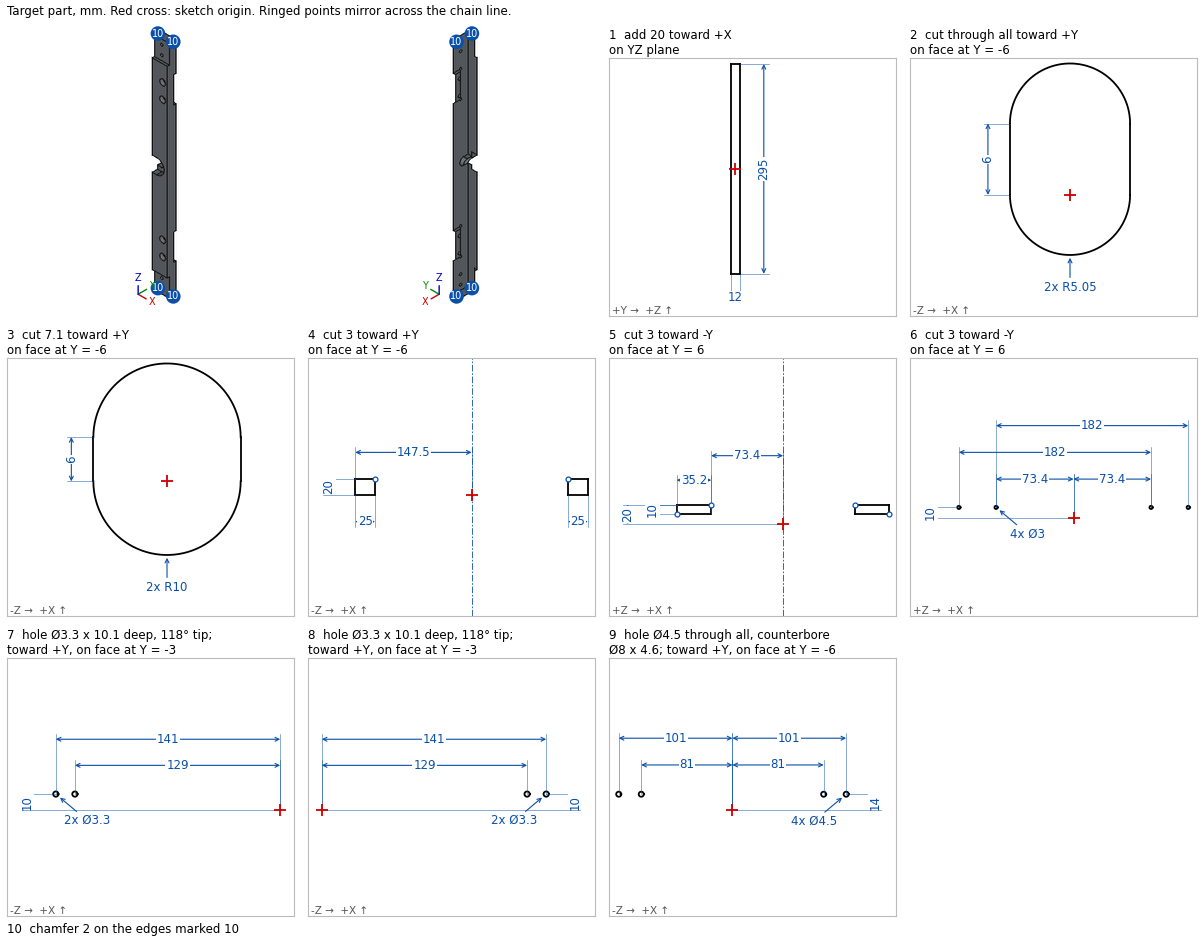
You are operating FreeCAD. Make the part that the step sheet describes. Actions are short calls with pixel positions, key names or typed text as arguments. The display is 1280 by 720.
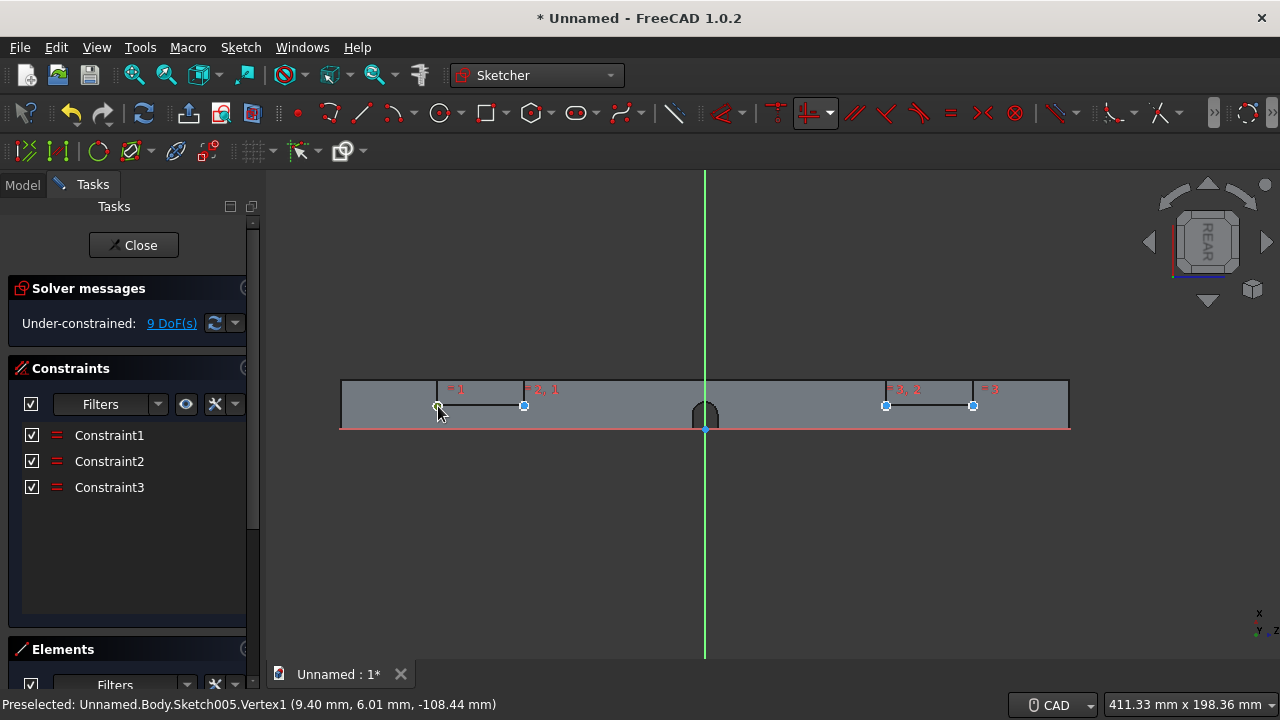
click(524, 406)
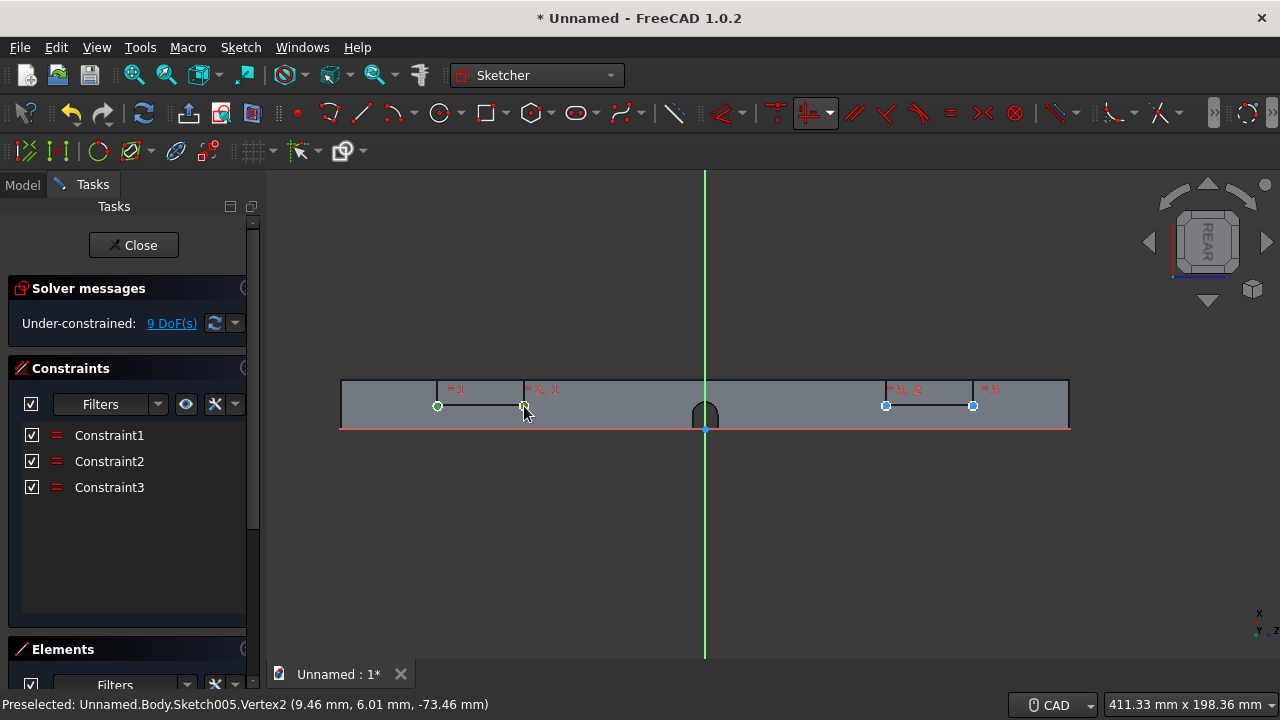
click(832, 114)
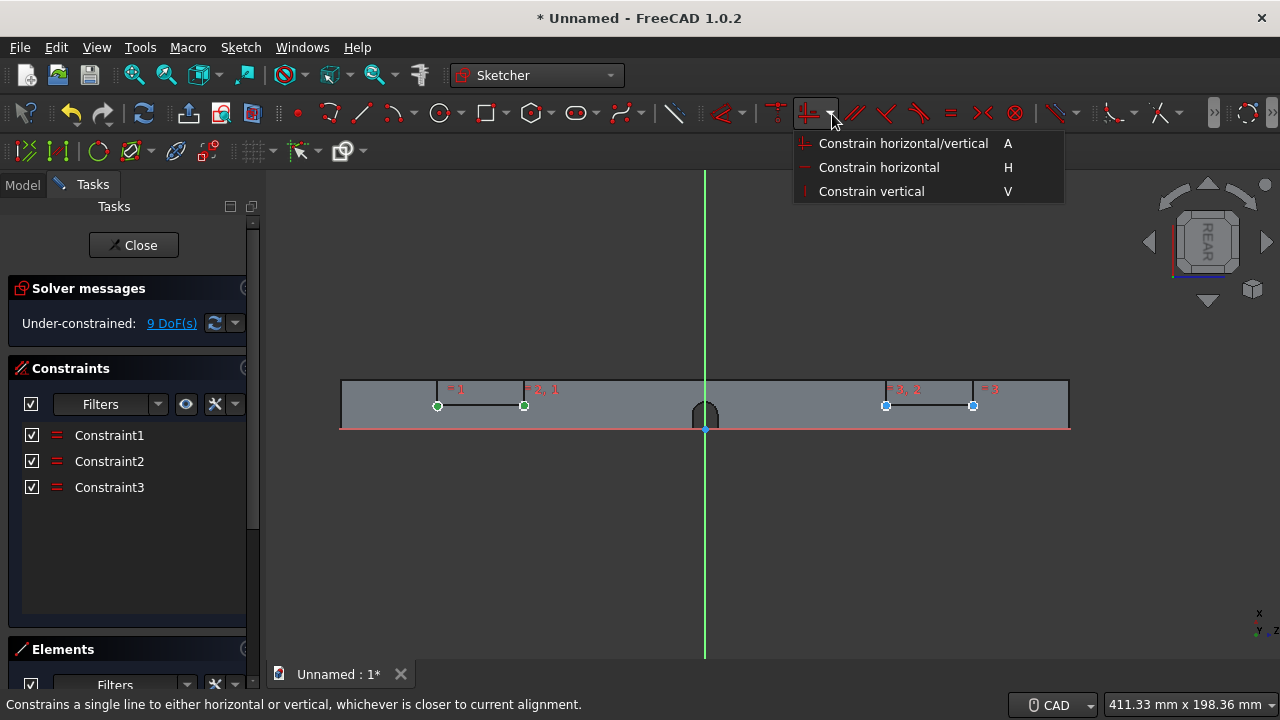
click(929, 167)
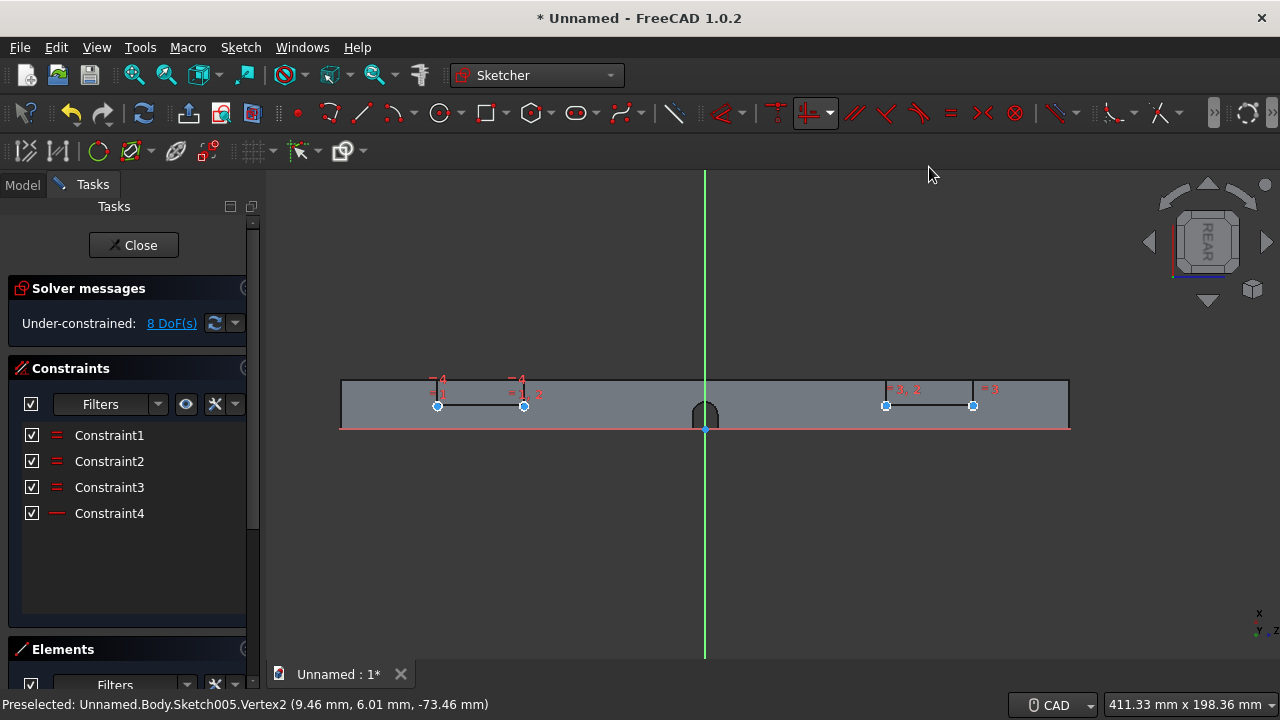
click(524, 406)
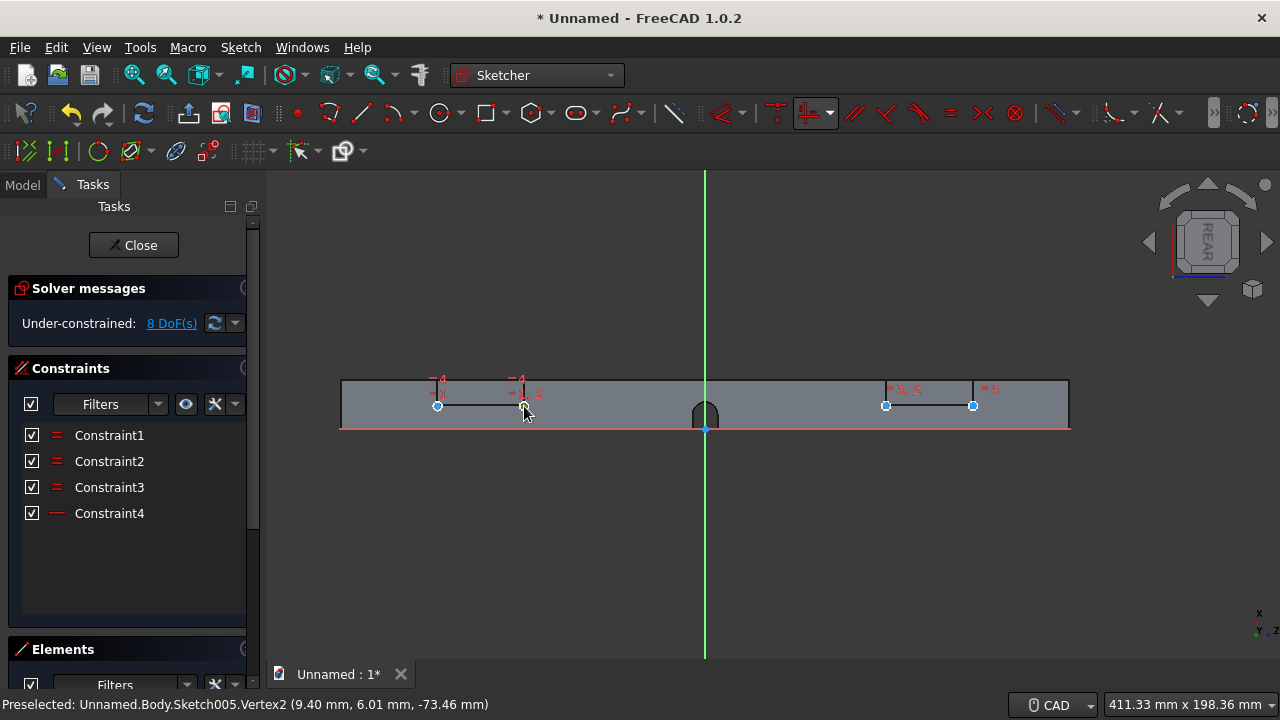
click(886, 406)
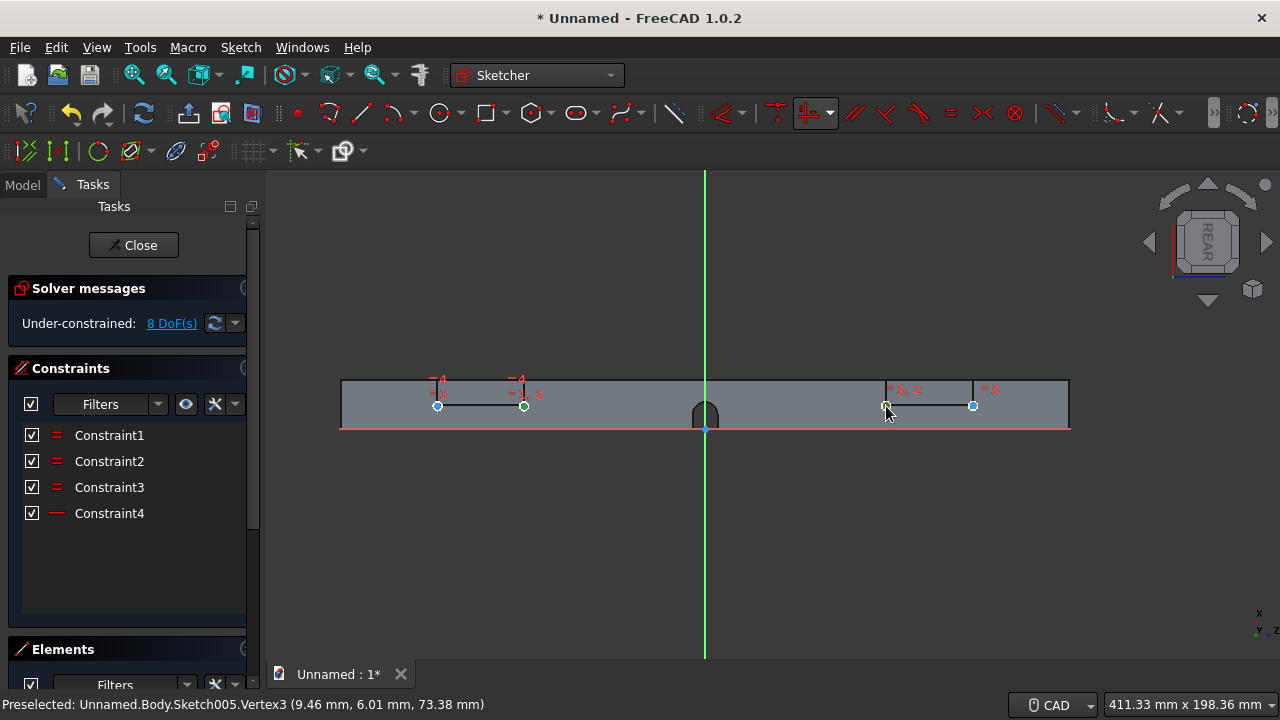
click(832, 114)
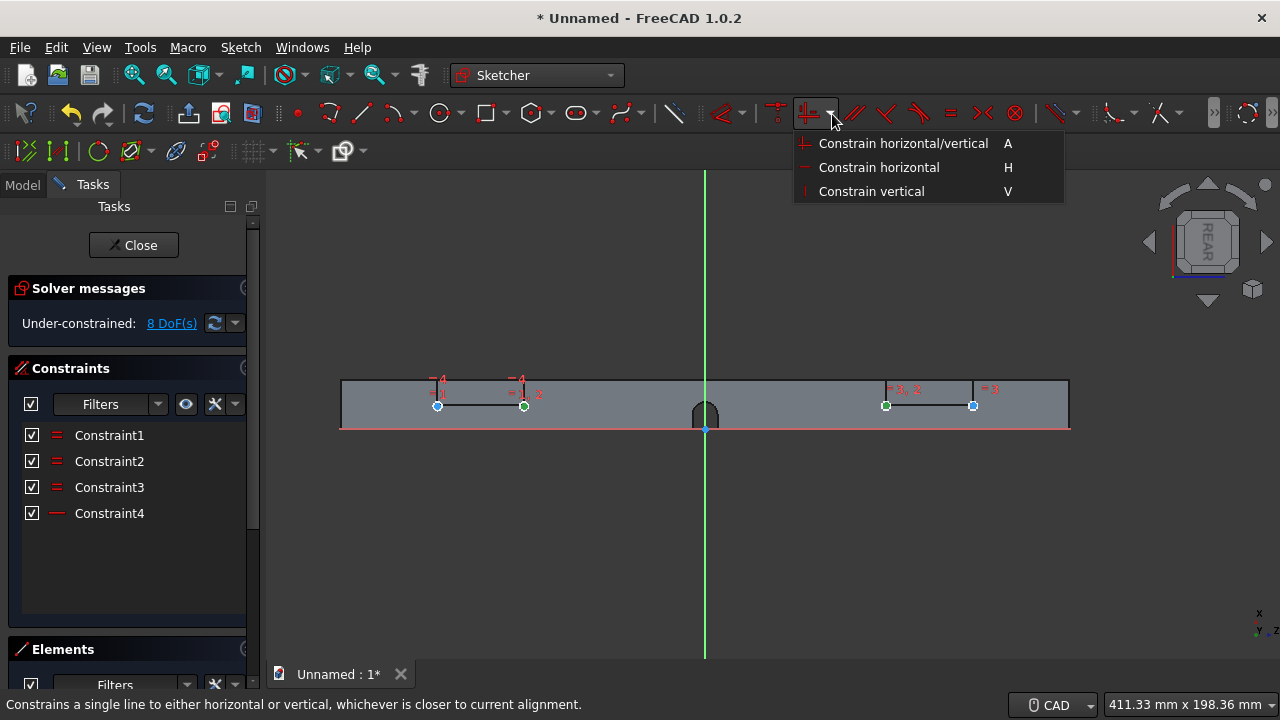
click(929, 167)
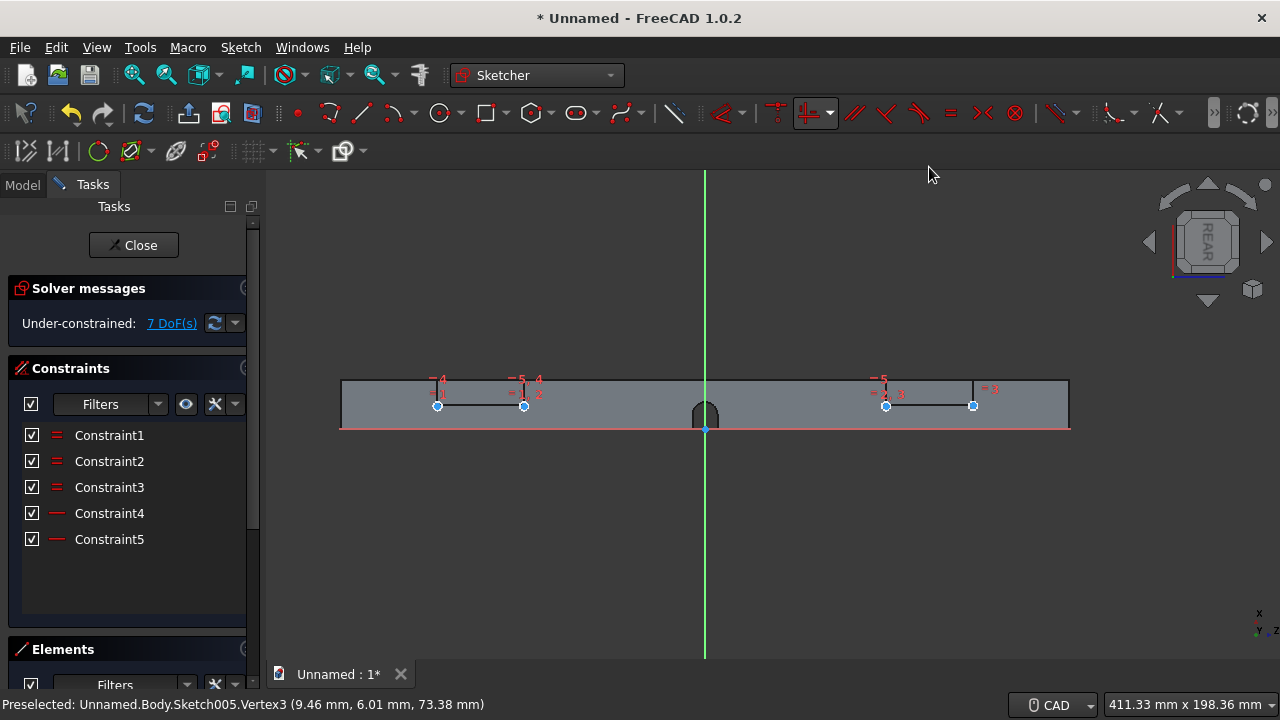
click(886, 406)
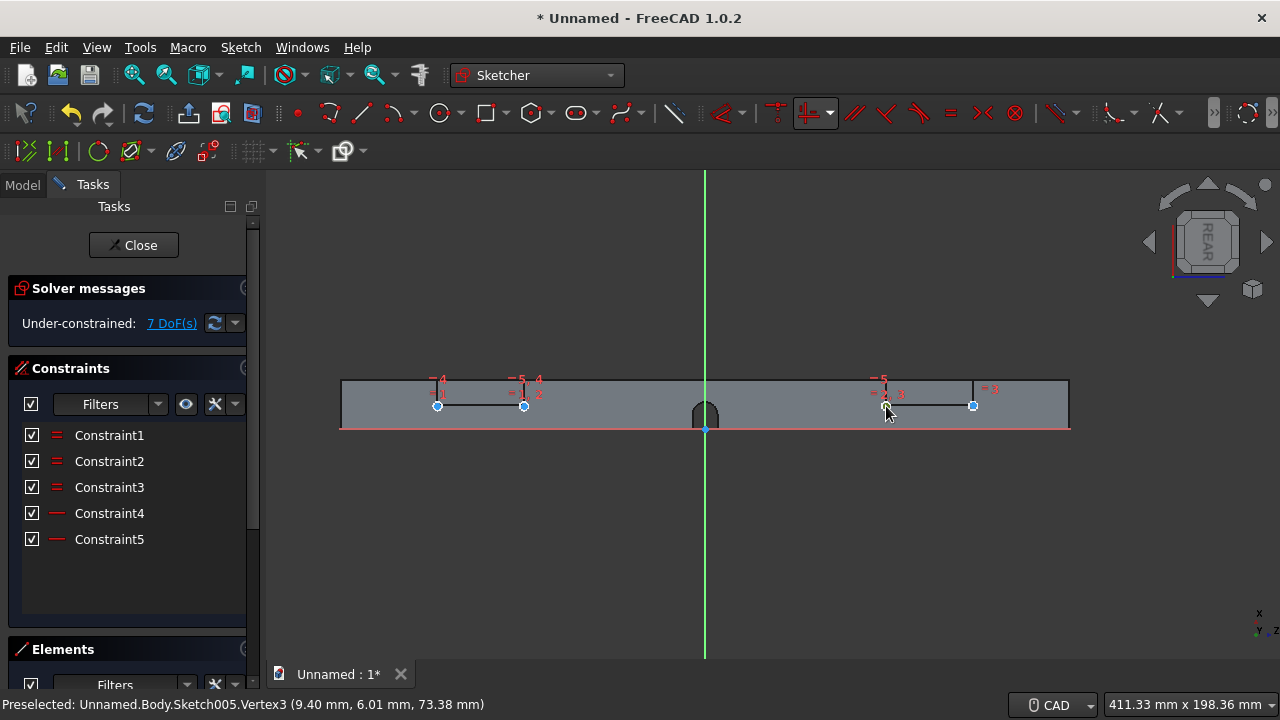
click(973, 406)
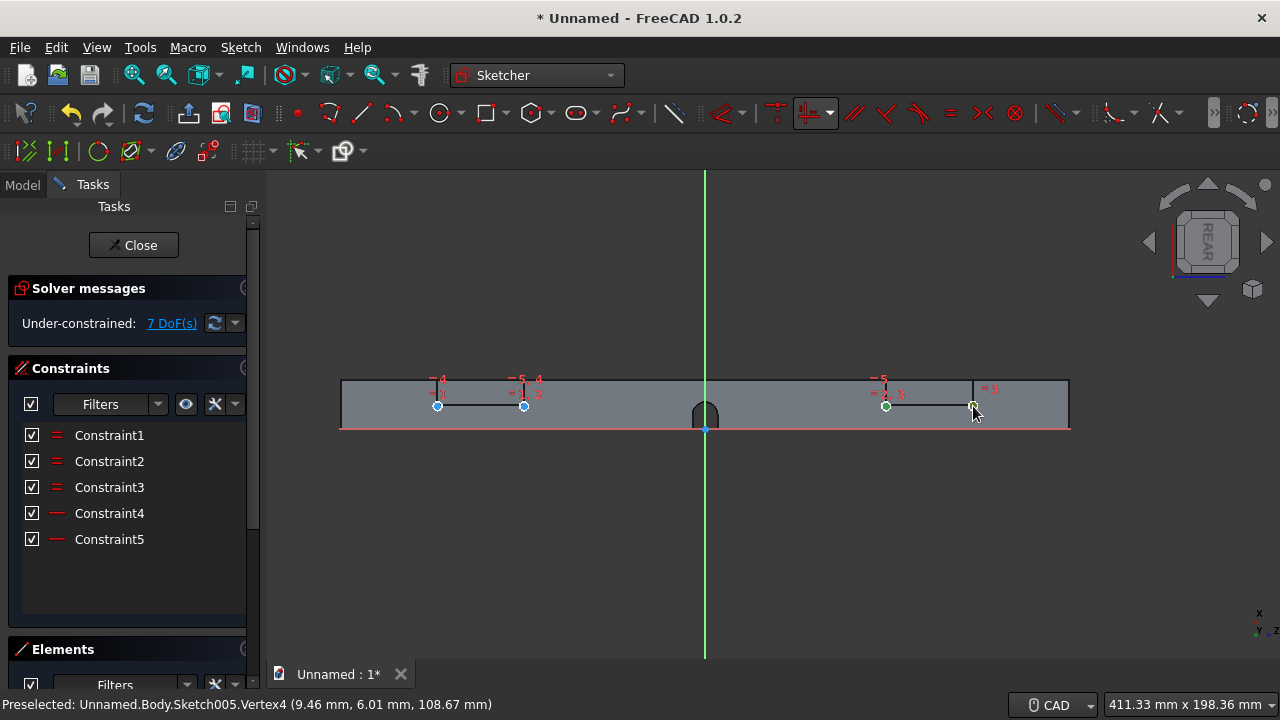
key(h)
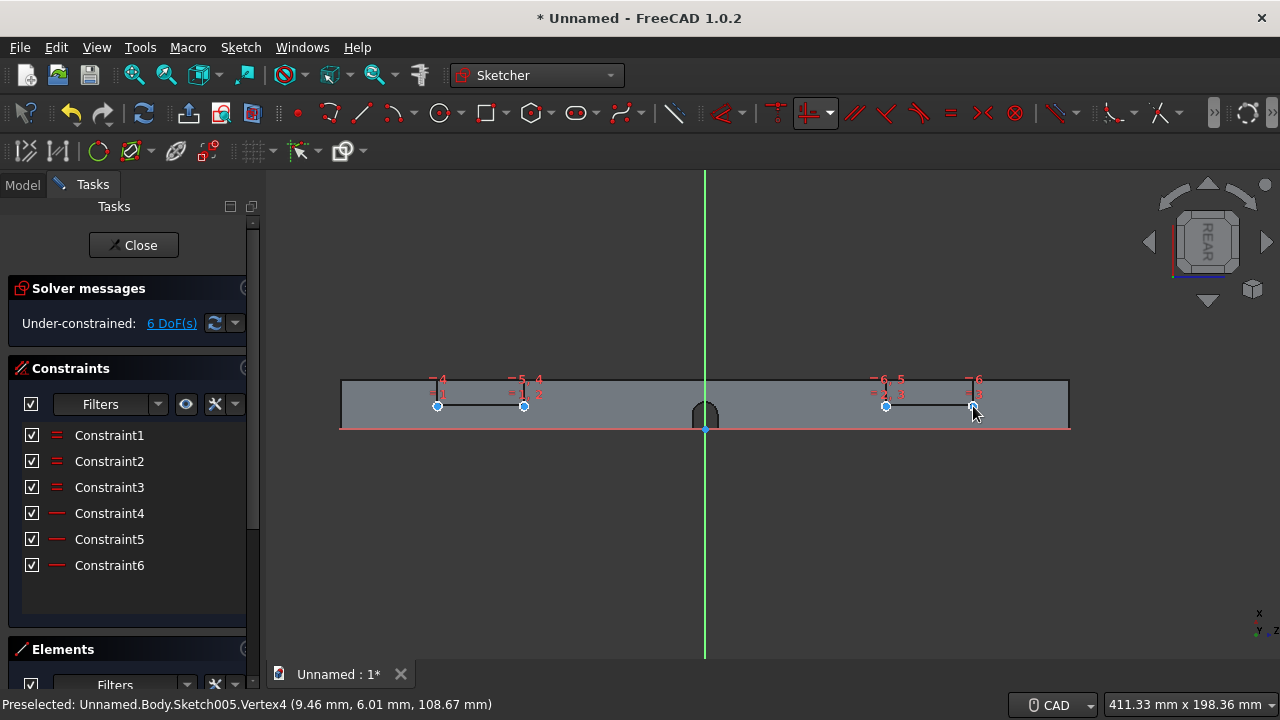
click(722, 114)